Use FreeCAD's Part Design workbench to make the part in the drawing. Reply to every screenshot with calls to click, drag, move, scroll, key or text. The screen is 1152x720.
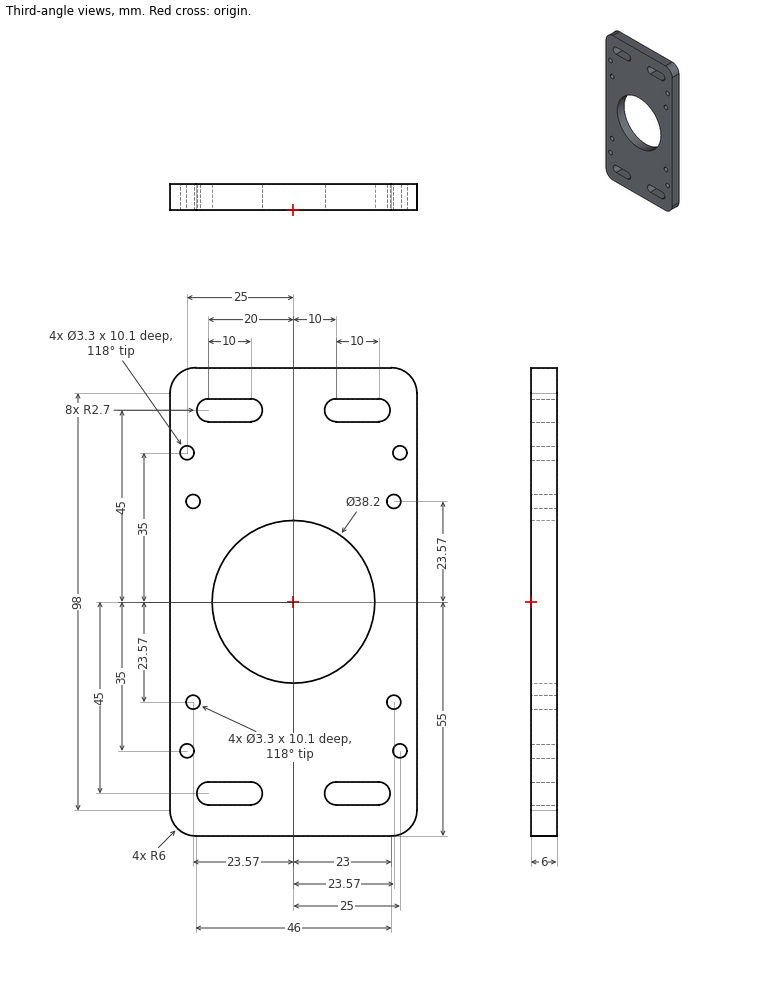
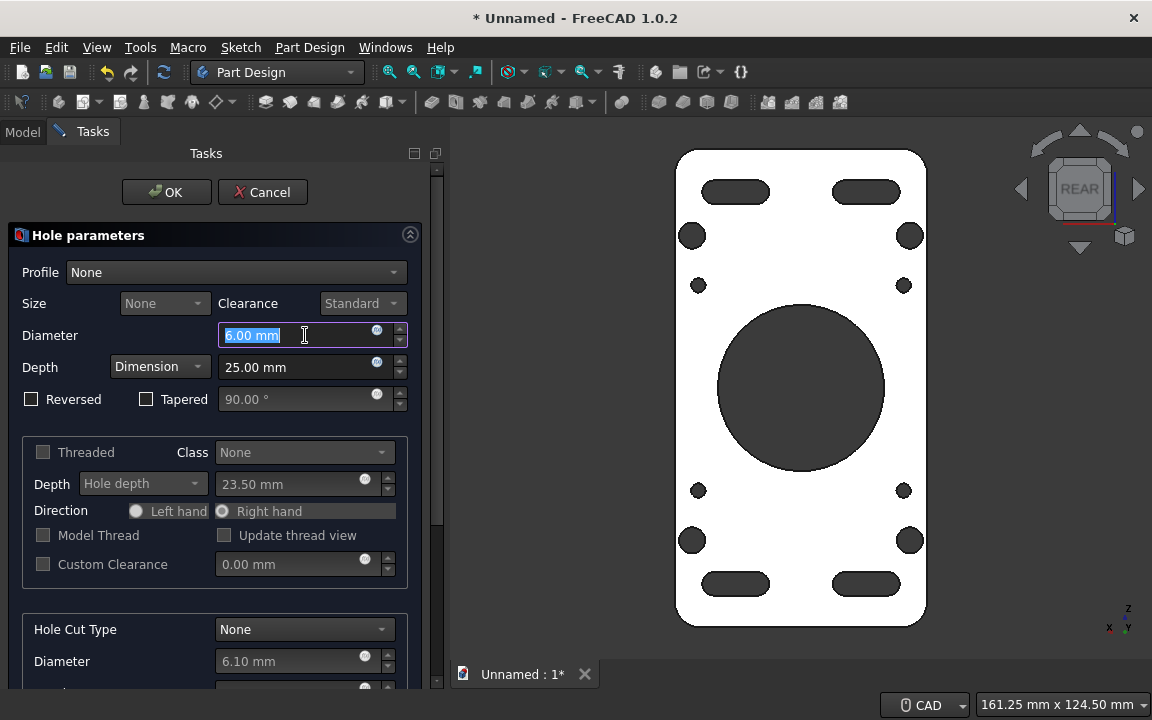
text(3.3)
key(Tab)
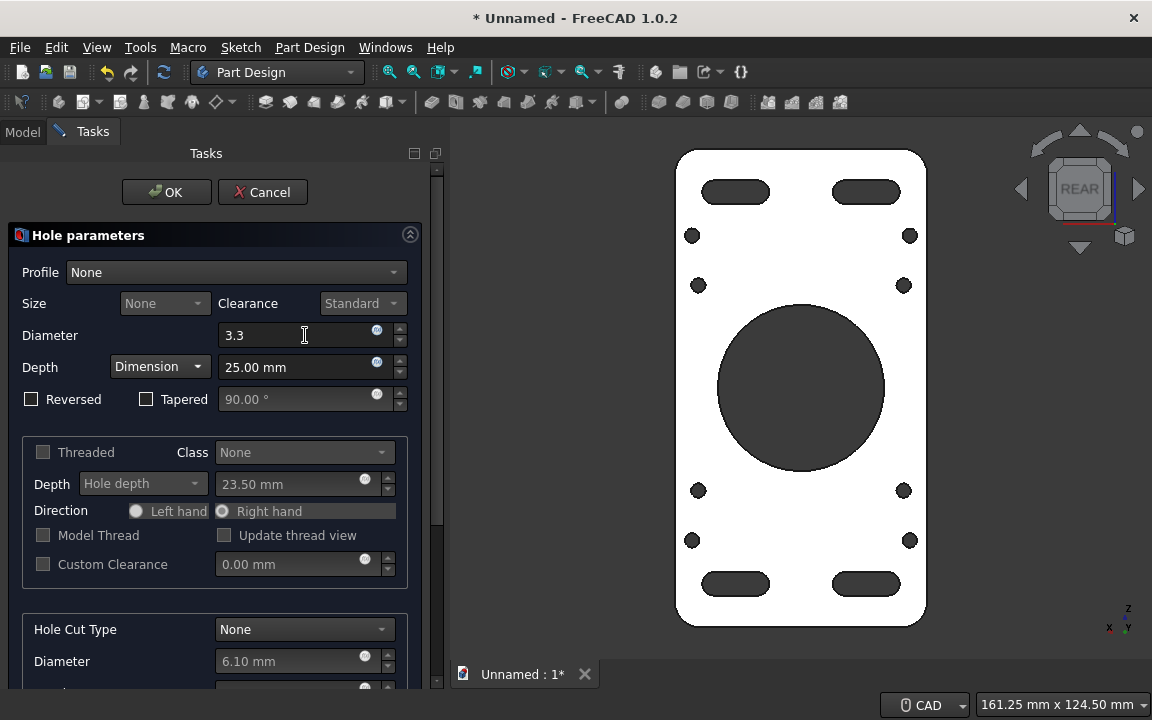
triple_click(305, 367)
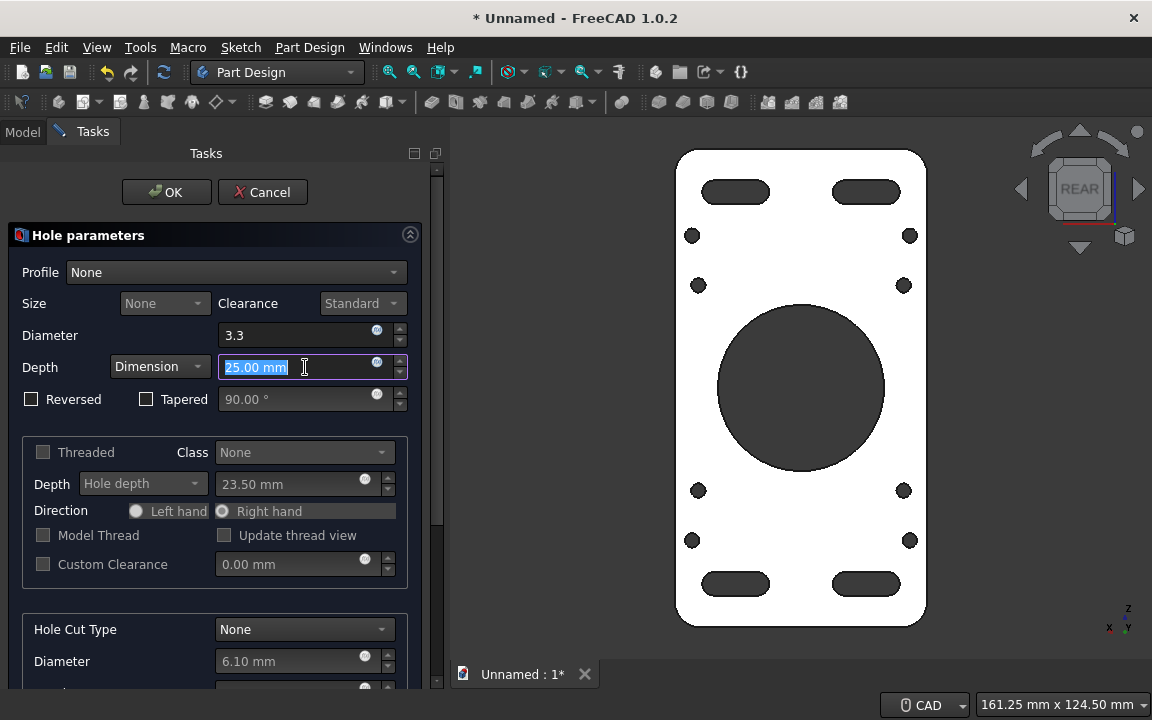
text(10.1)
key(Tab)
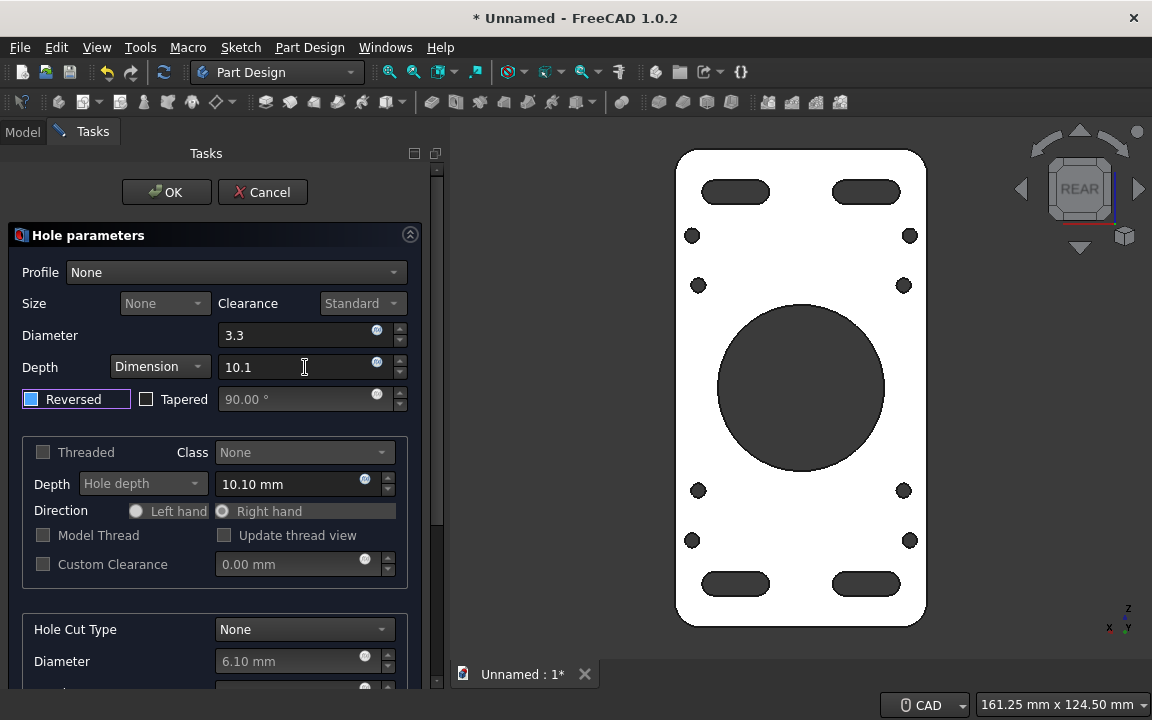
click(167, 192)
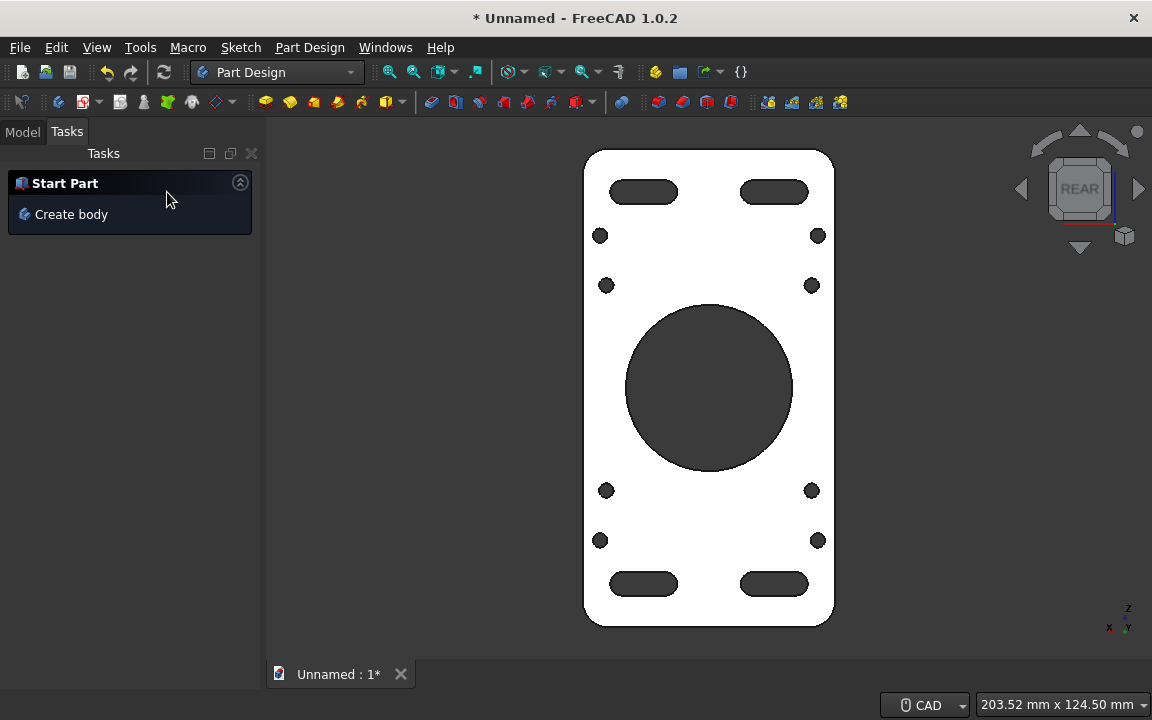
key(0)